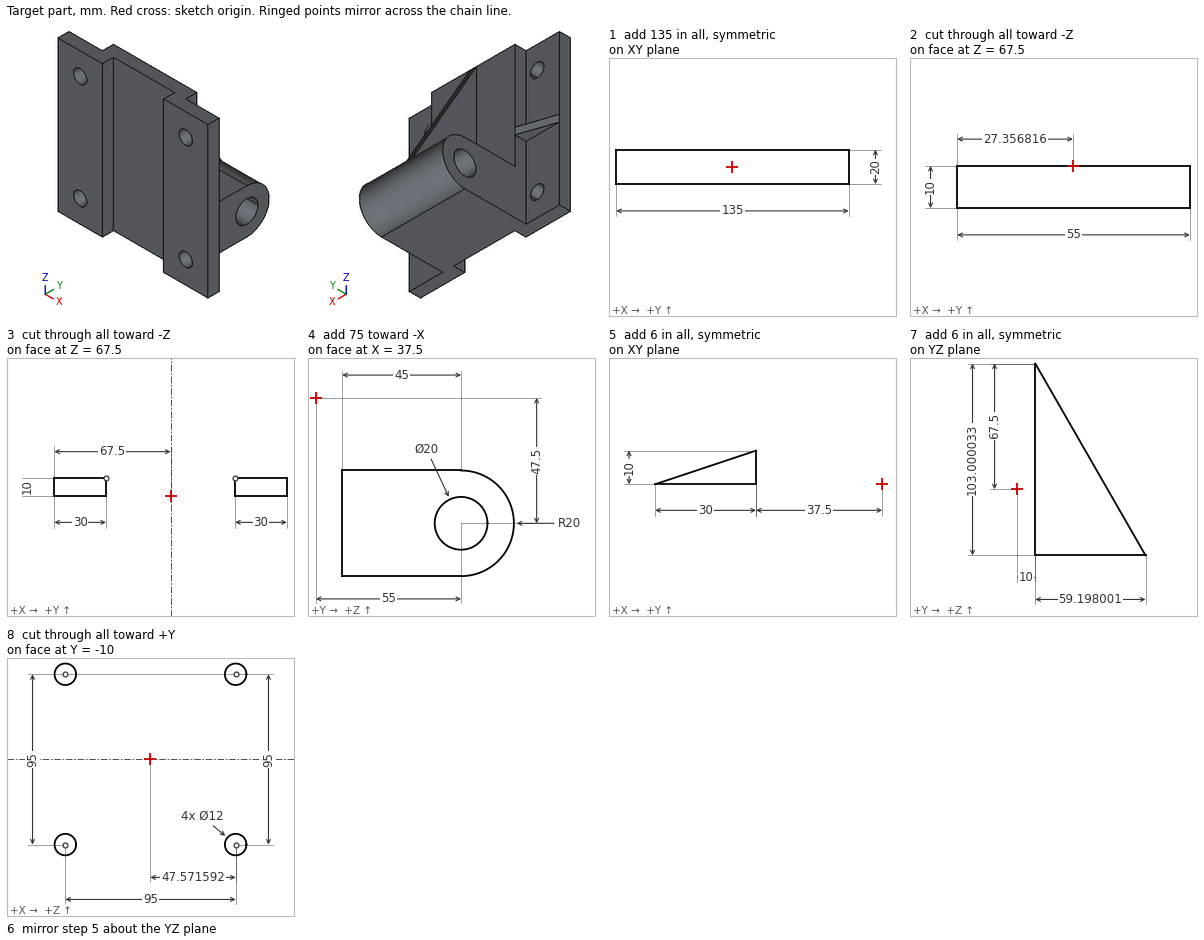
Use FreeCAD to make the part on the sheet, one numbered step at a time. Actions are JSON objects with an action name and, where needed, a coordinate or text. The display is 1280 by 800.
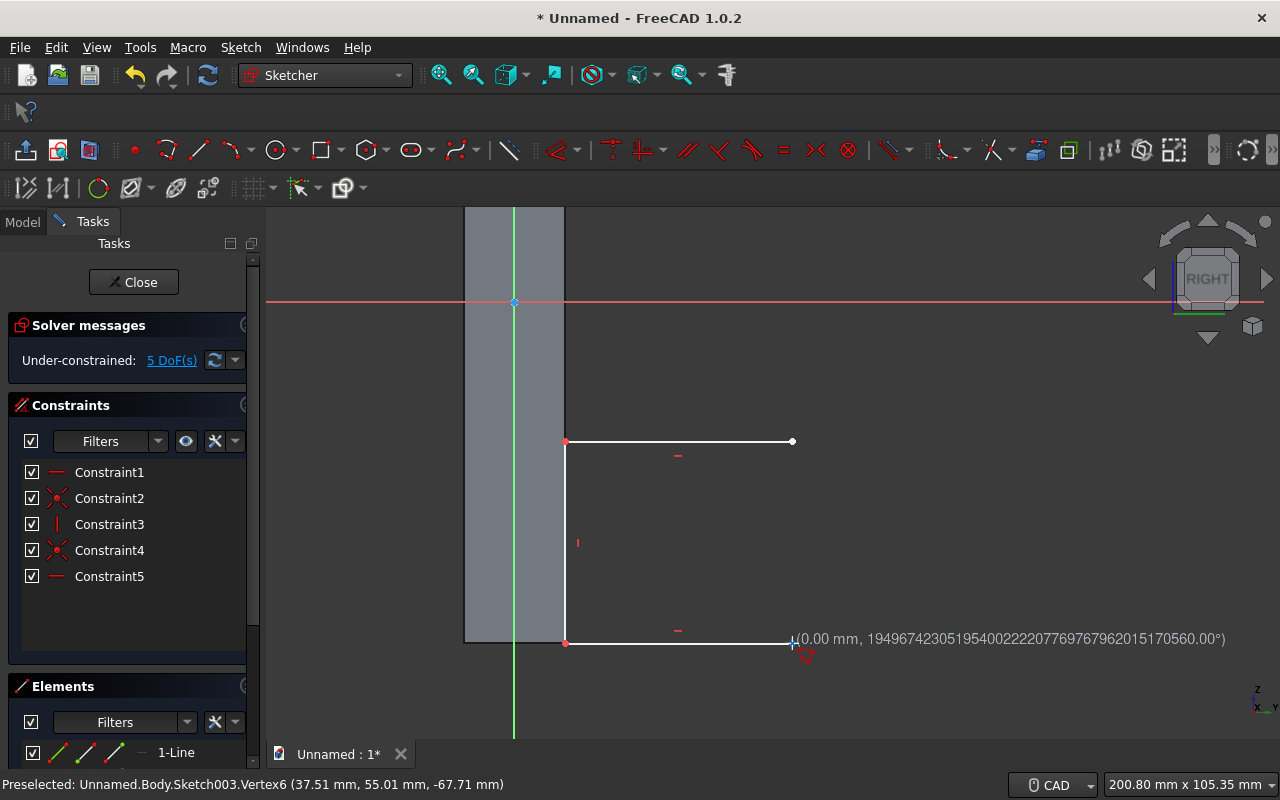
{"action": "left_click", "coordinate": [232, 150]}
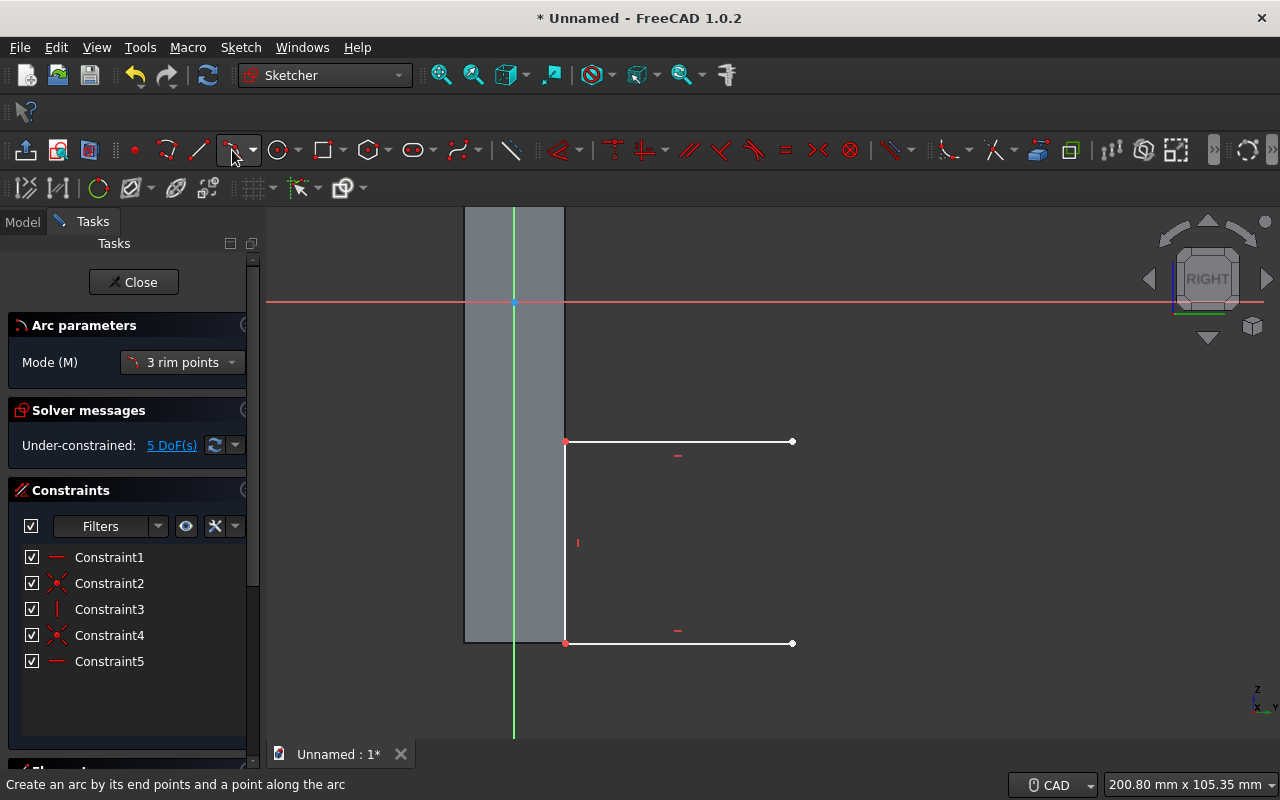
{"action": "left_click", "coordinate": [792, 644]}
{"action": "left_click", "coordinate": [792, 442]}
{"action": "left_click", "coordinate": [893, 542]}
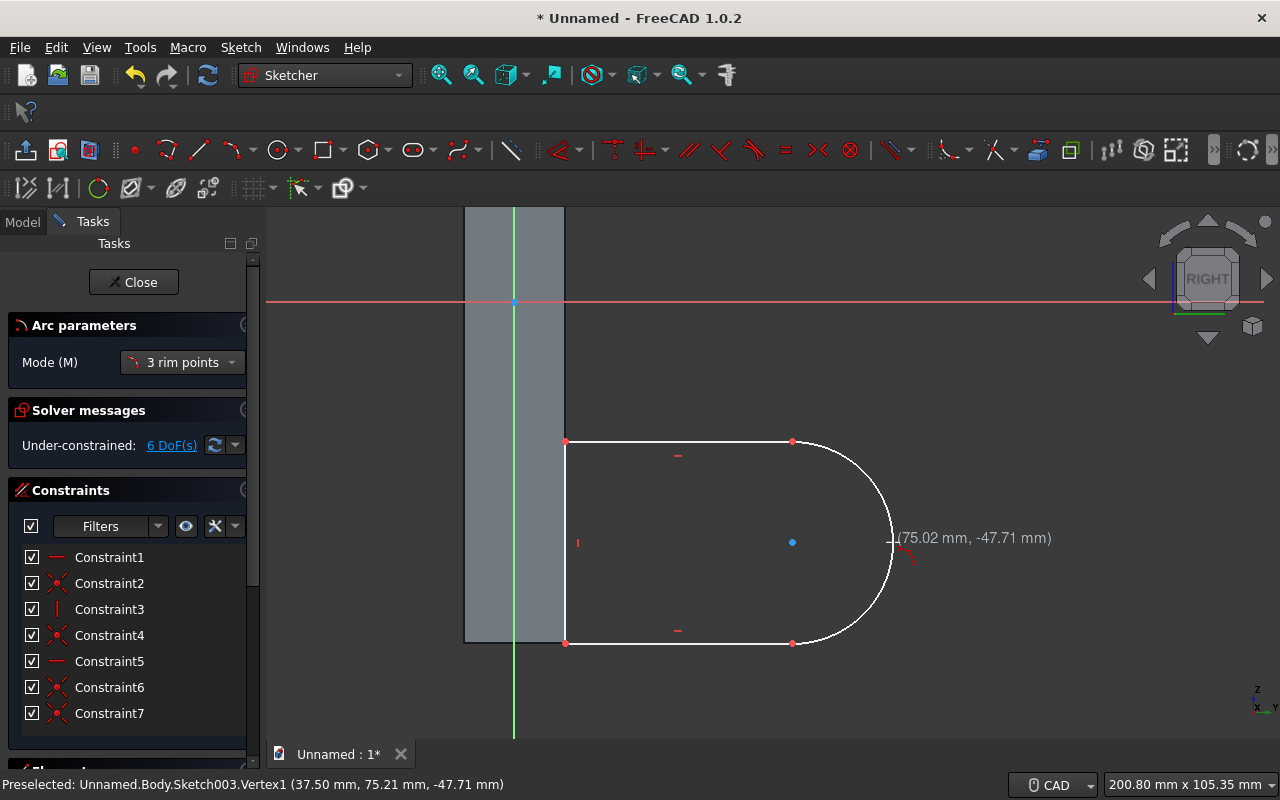
{"action": "left_click", "coordinate": [278, 150]}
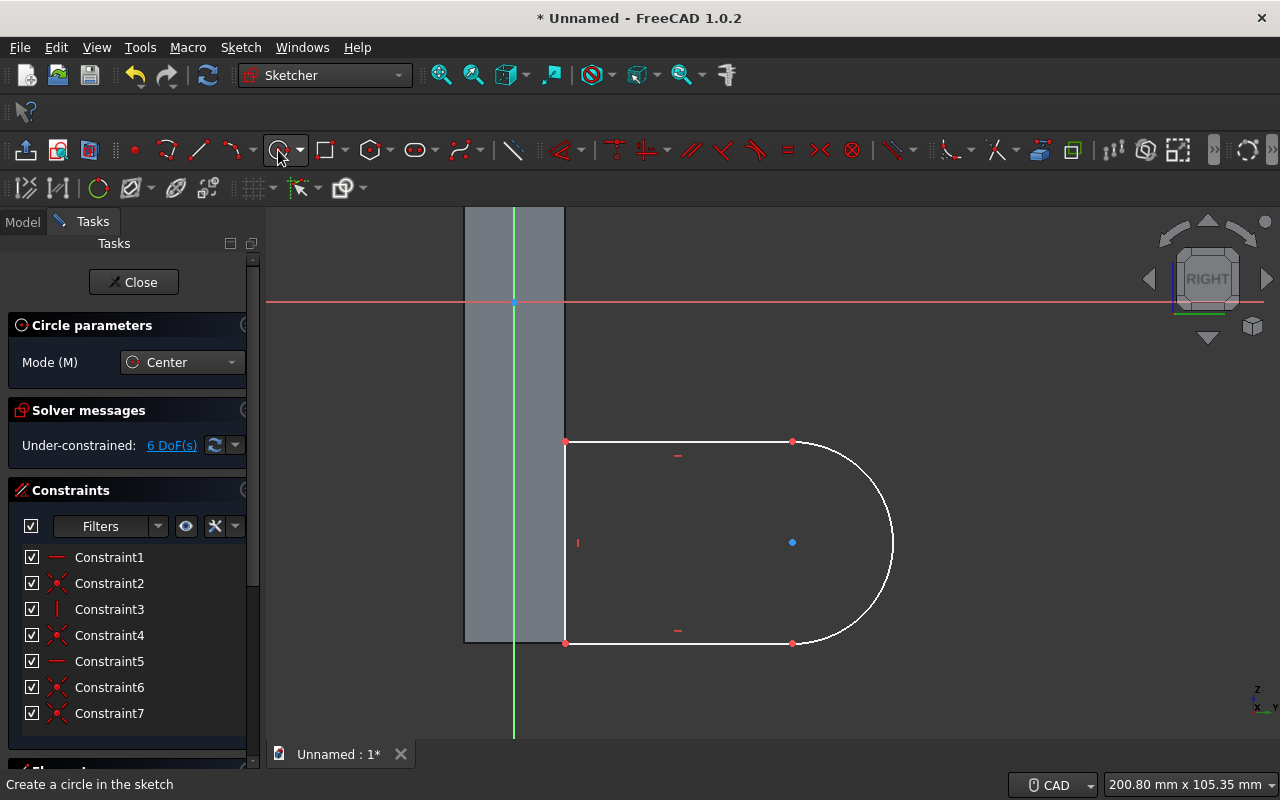
{"action": "left_click", "coordinate": [792, 542]}
{"action": "left_click", "coordinate": [828, 506]}
{"action": "key", "text": "Escape"}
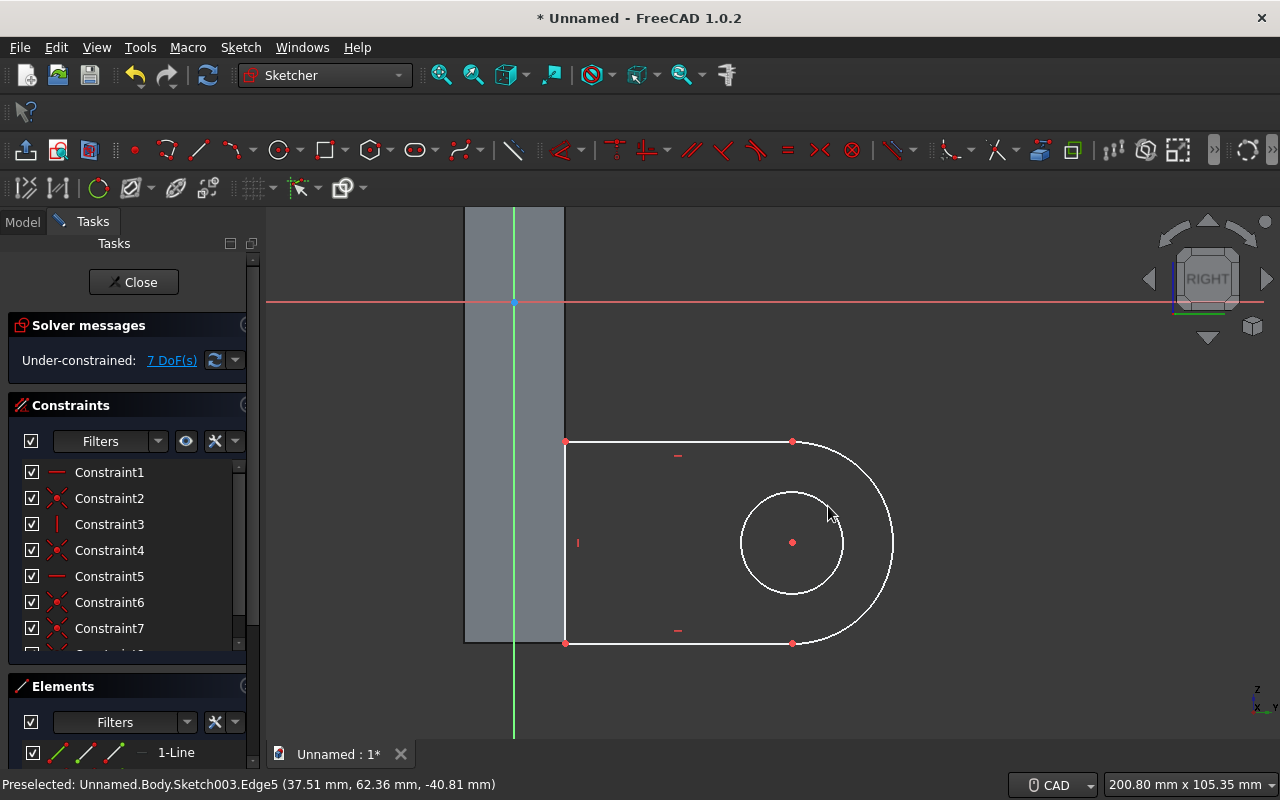
{"action": "left_click", "coordinate": [724, 442]}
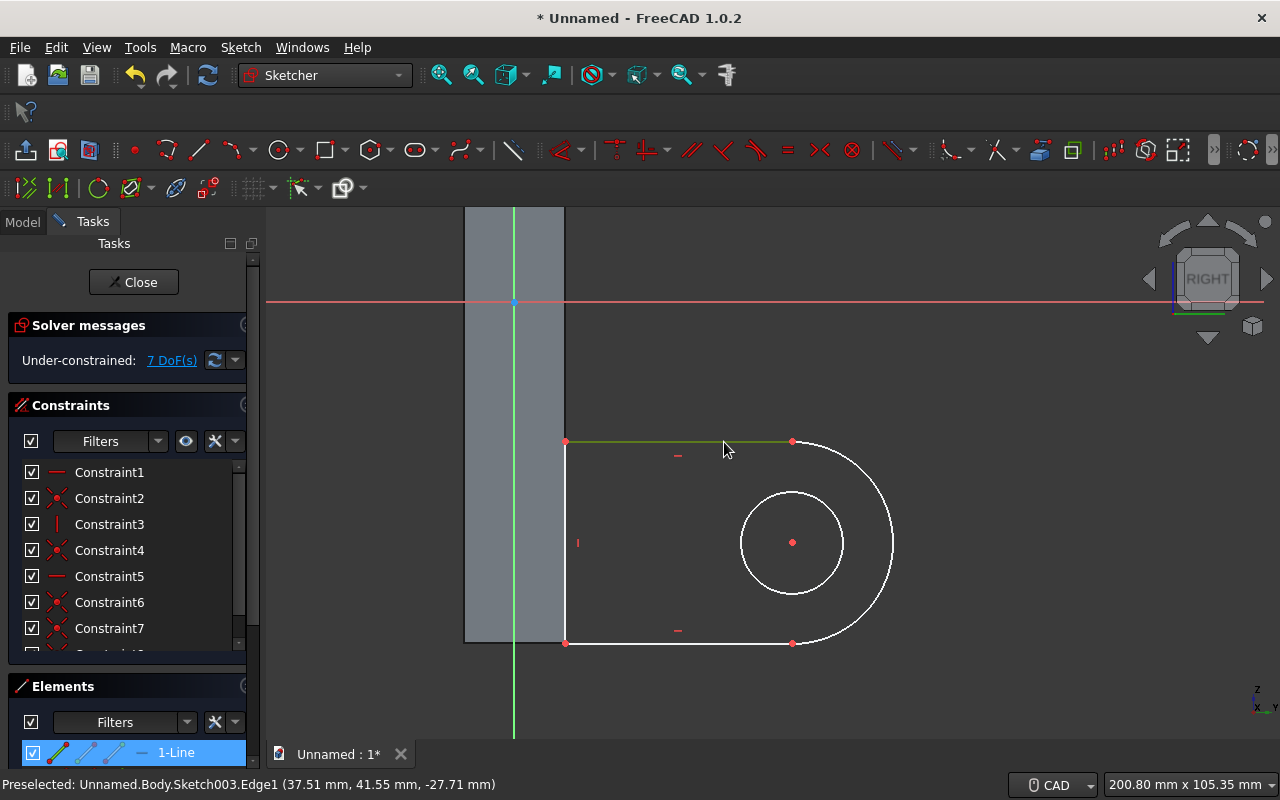
{"action": "left_click", "coordinate": [874, 602]}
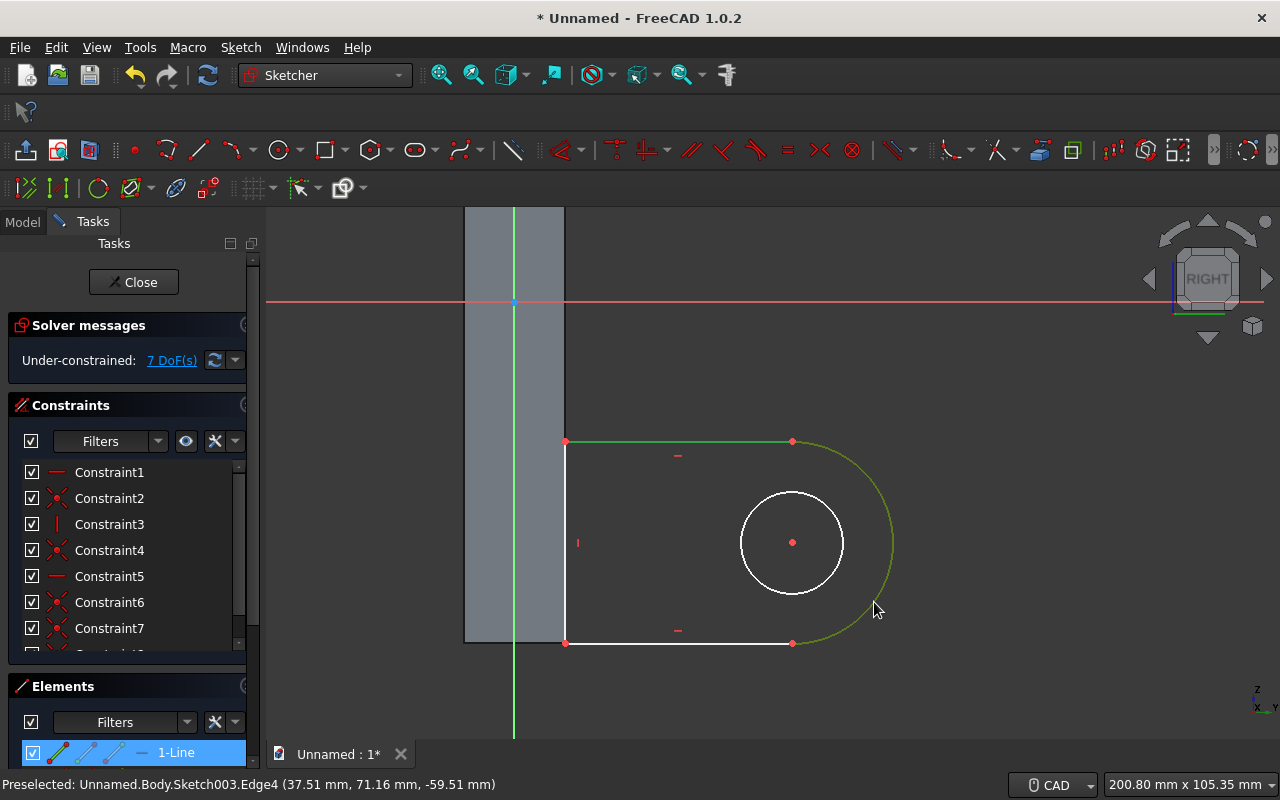
{"action": "left_click", "coordinate": [756, 150]}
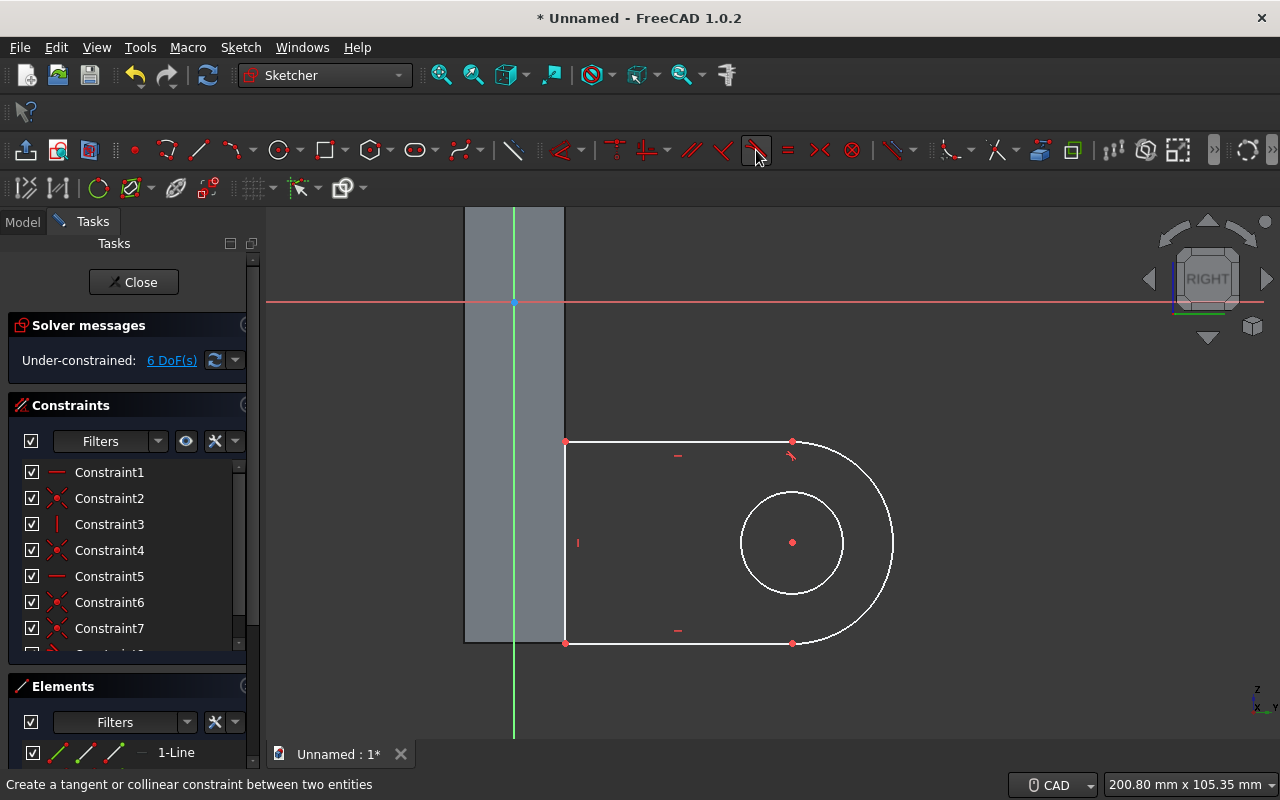
{"action": "left_click", "coordinate": [633, 644]}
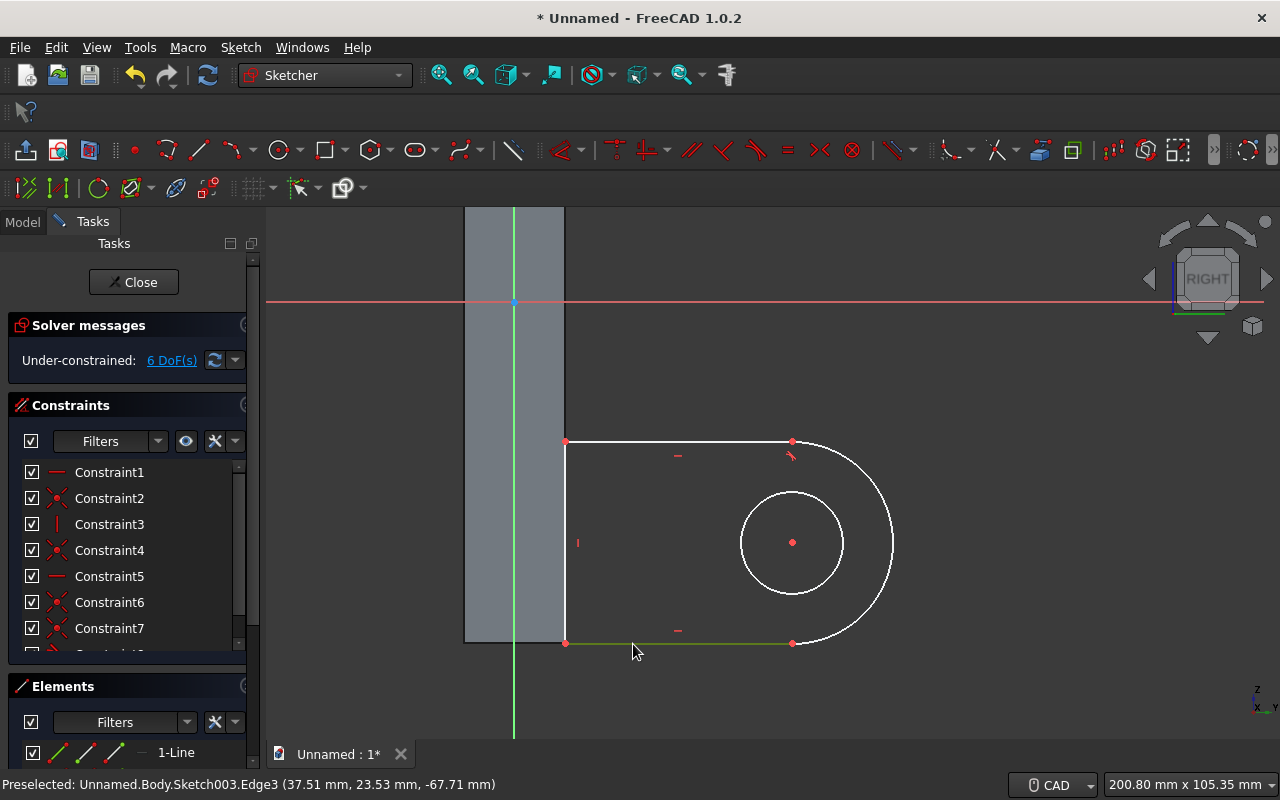
{"action": "left_click", "coordinate": [874, 602]}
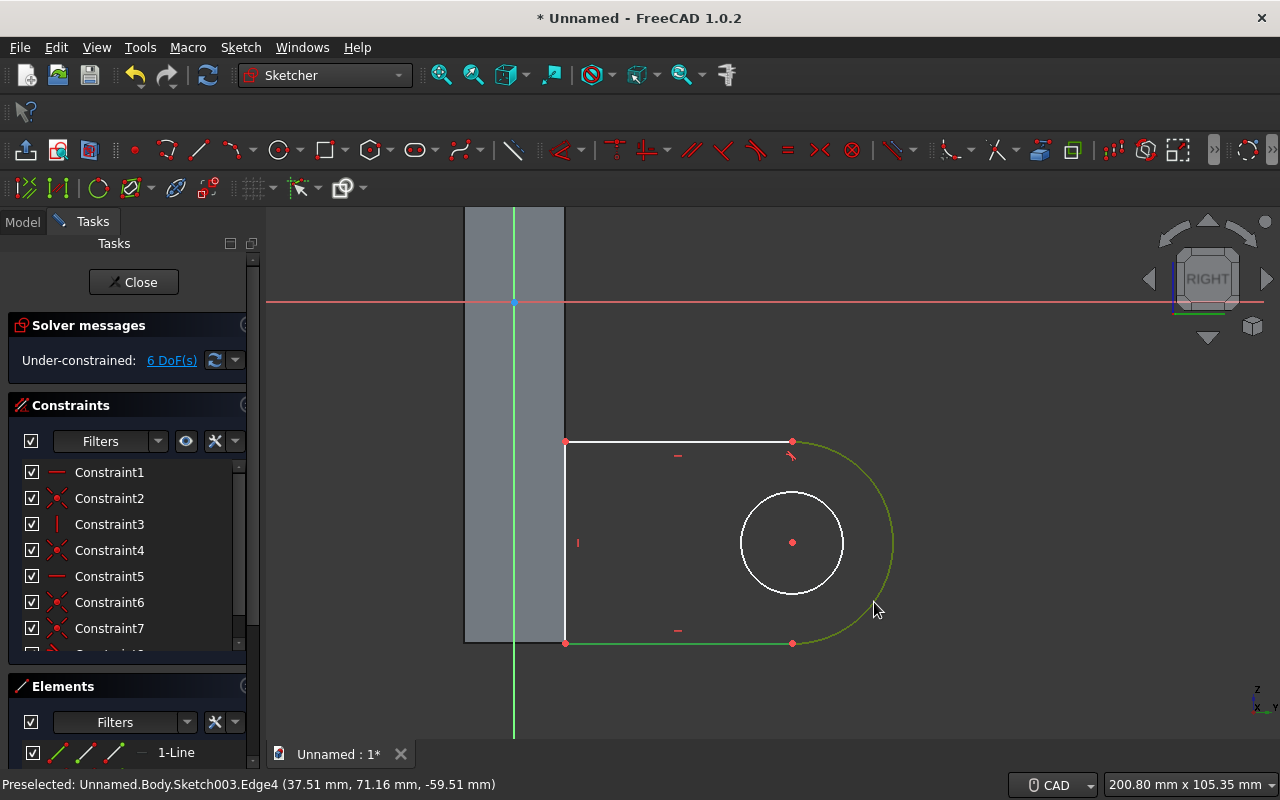
{"action": "key", "text": "t"}